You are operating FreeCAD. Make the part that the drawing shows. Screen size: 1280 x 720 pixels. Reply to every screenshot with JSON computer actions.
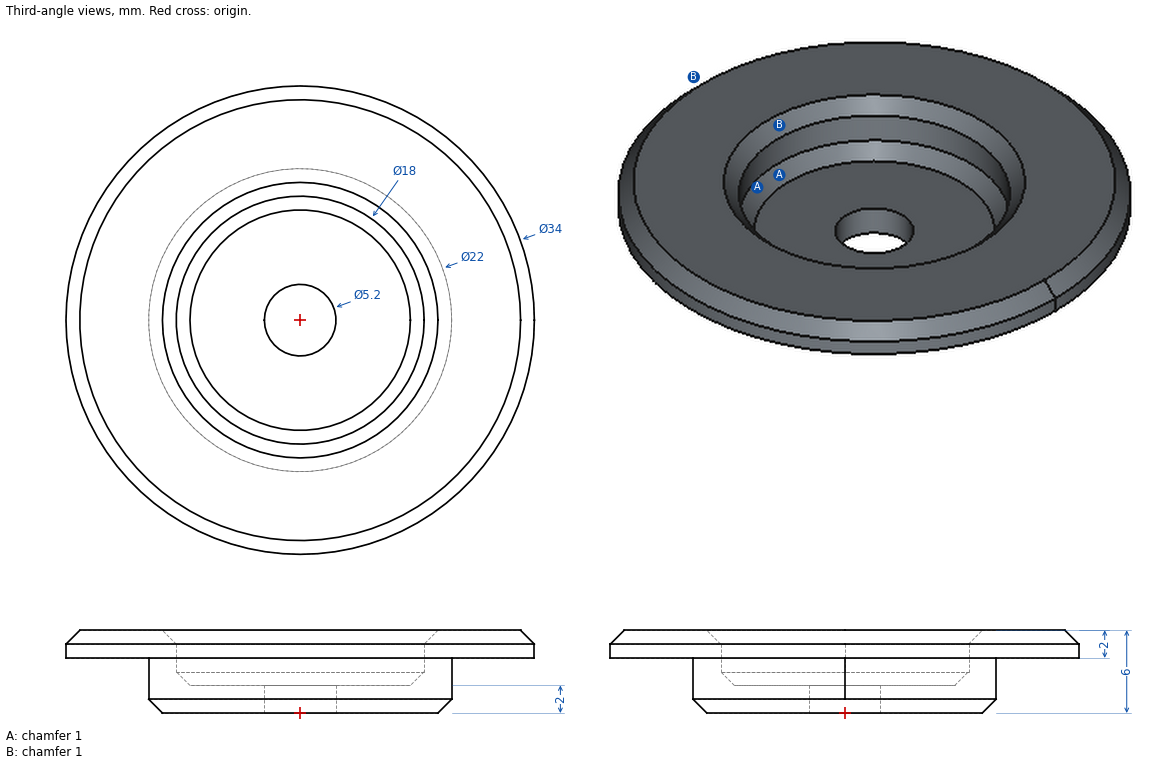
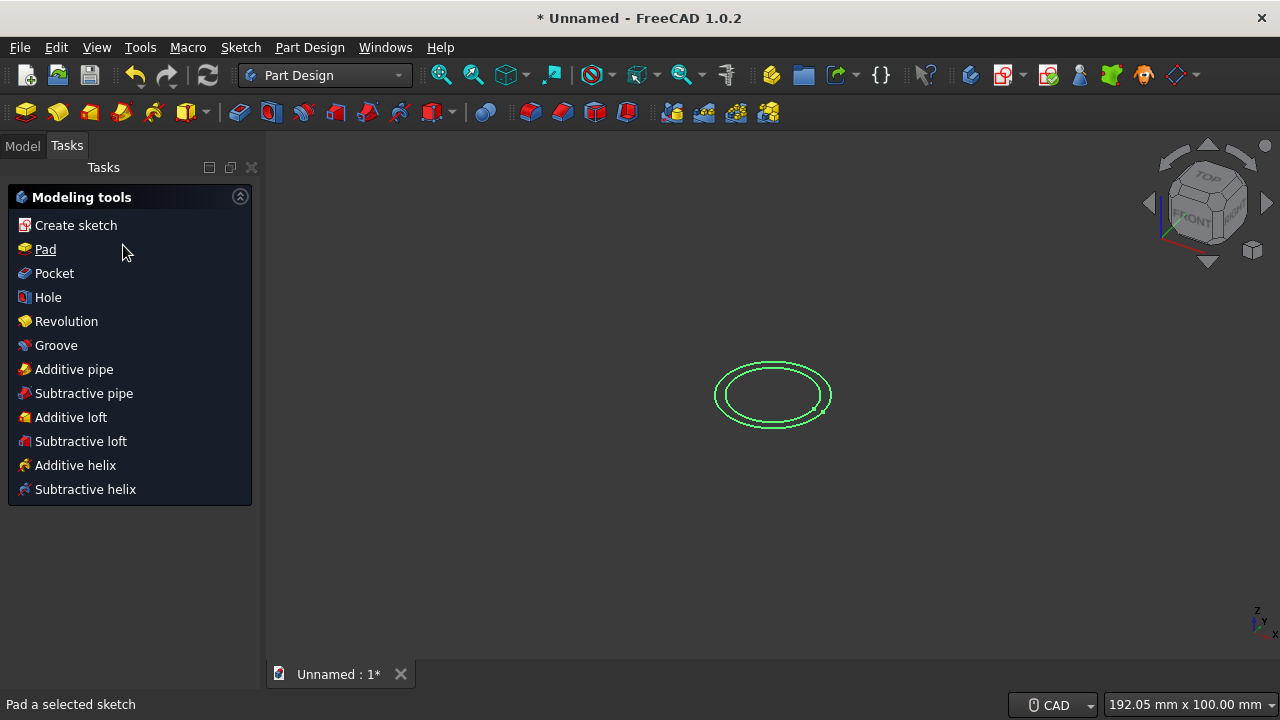
{"action": "left_click", "coordinate": [26, 112]}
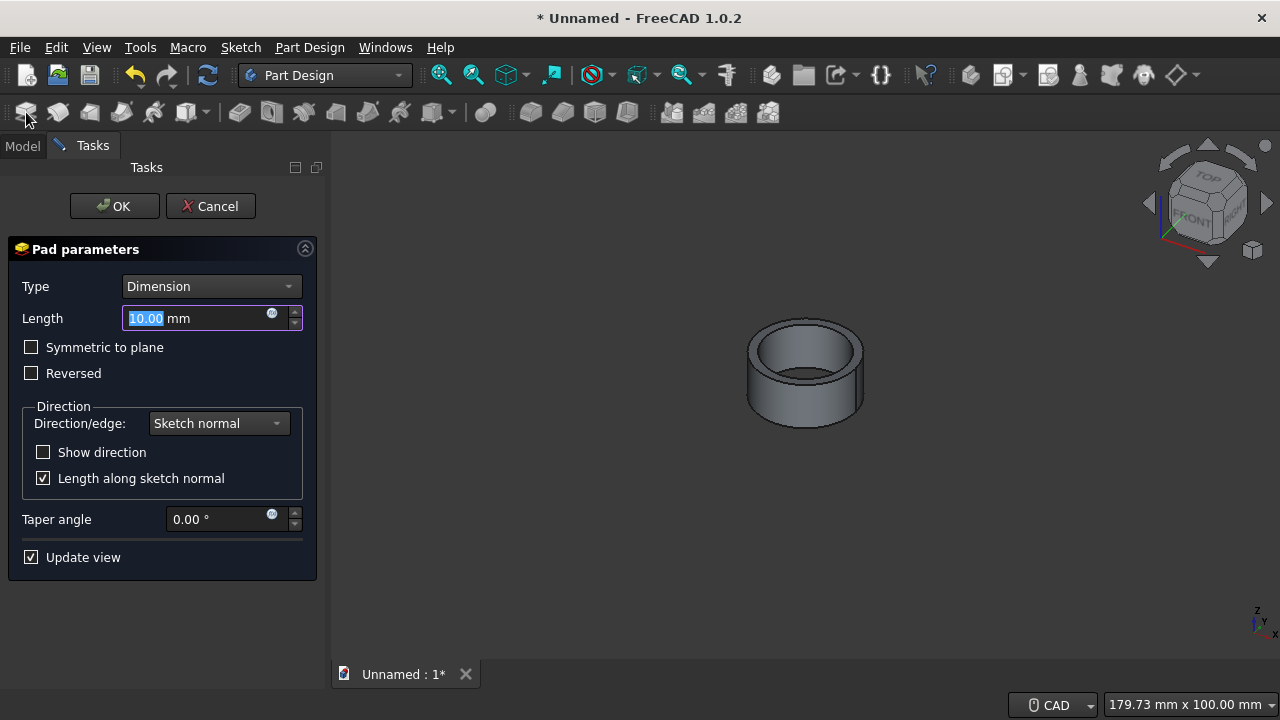
{"action": "type", "text": "6"}
{"action": "key", "text": "Tab"}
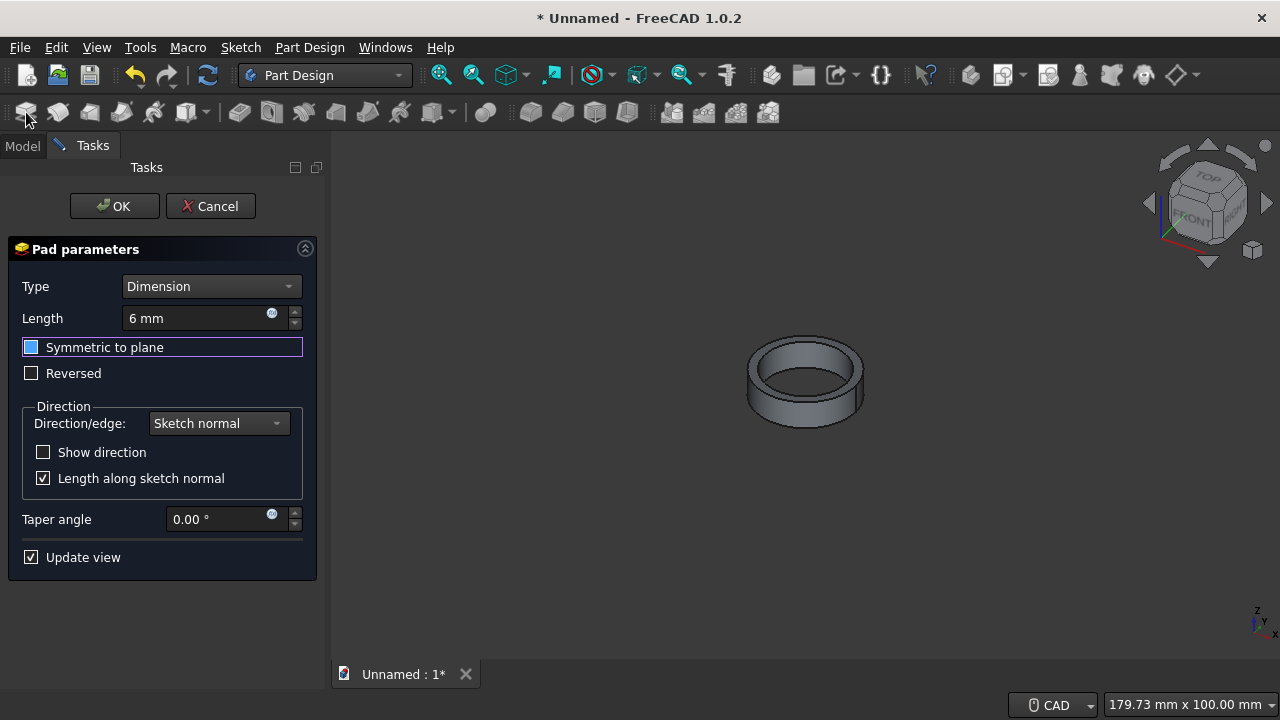
{"action": "left_click", "coordinate": [115, 206]}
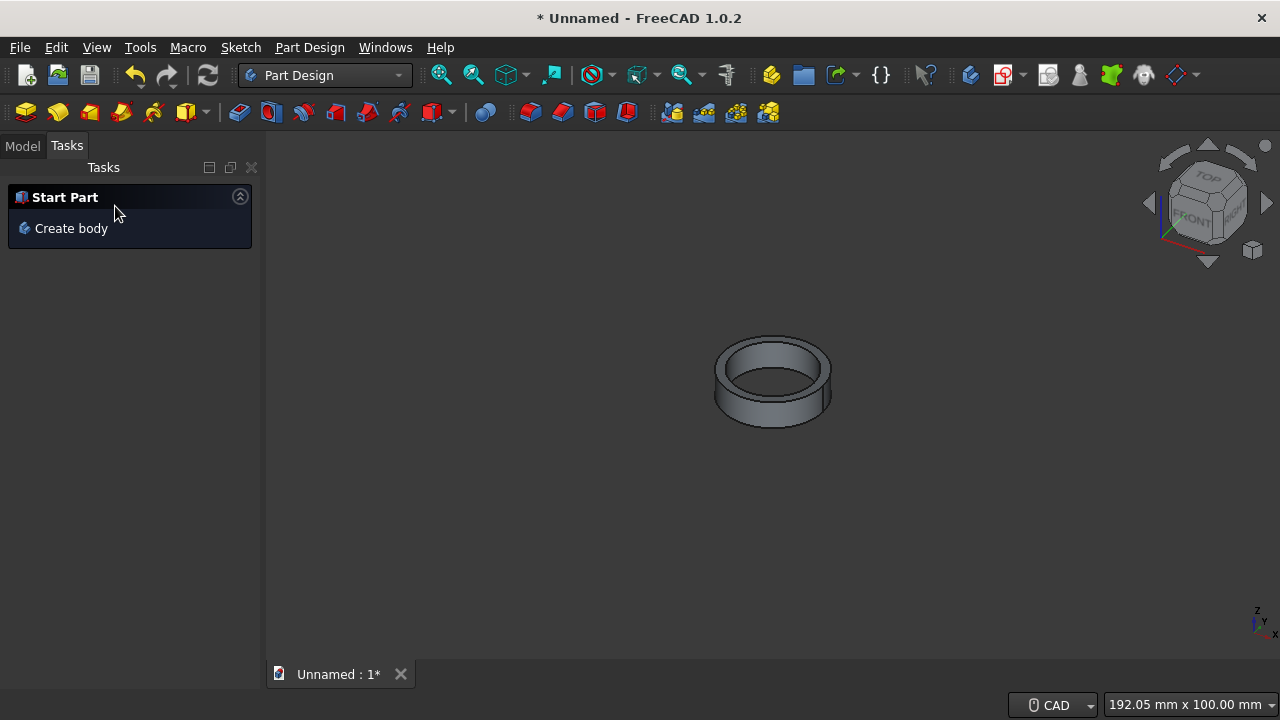
{"action": "left_click", "coordinate": [442, 76]}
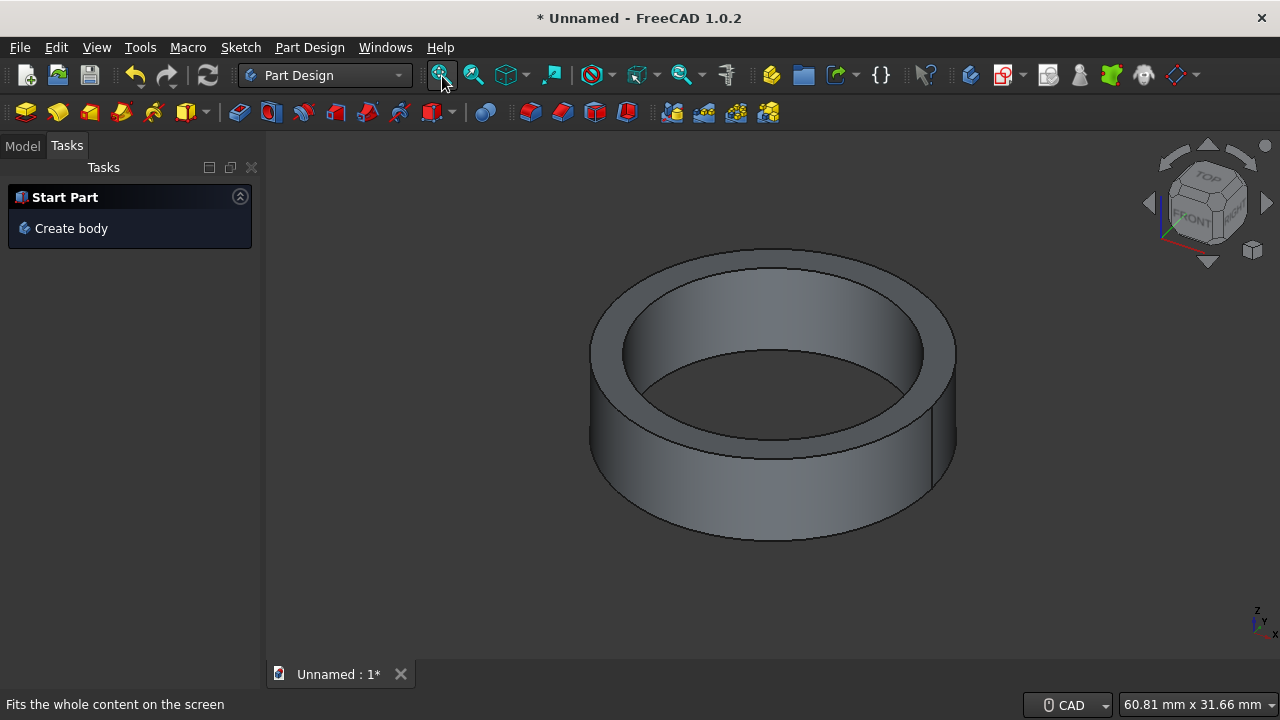
{"action": "key", "text": "5"}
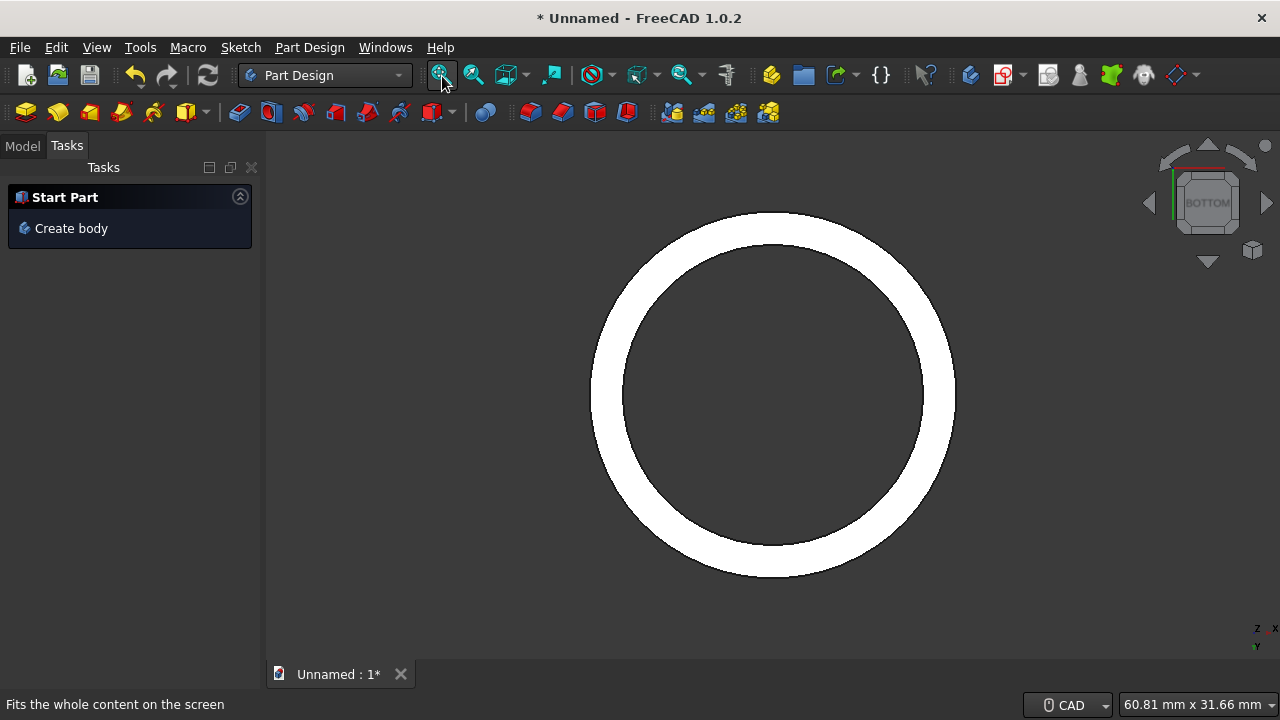
{"action": "left_click", "coordinate": [721, 237]}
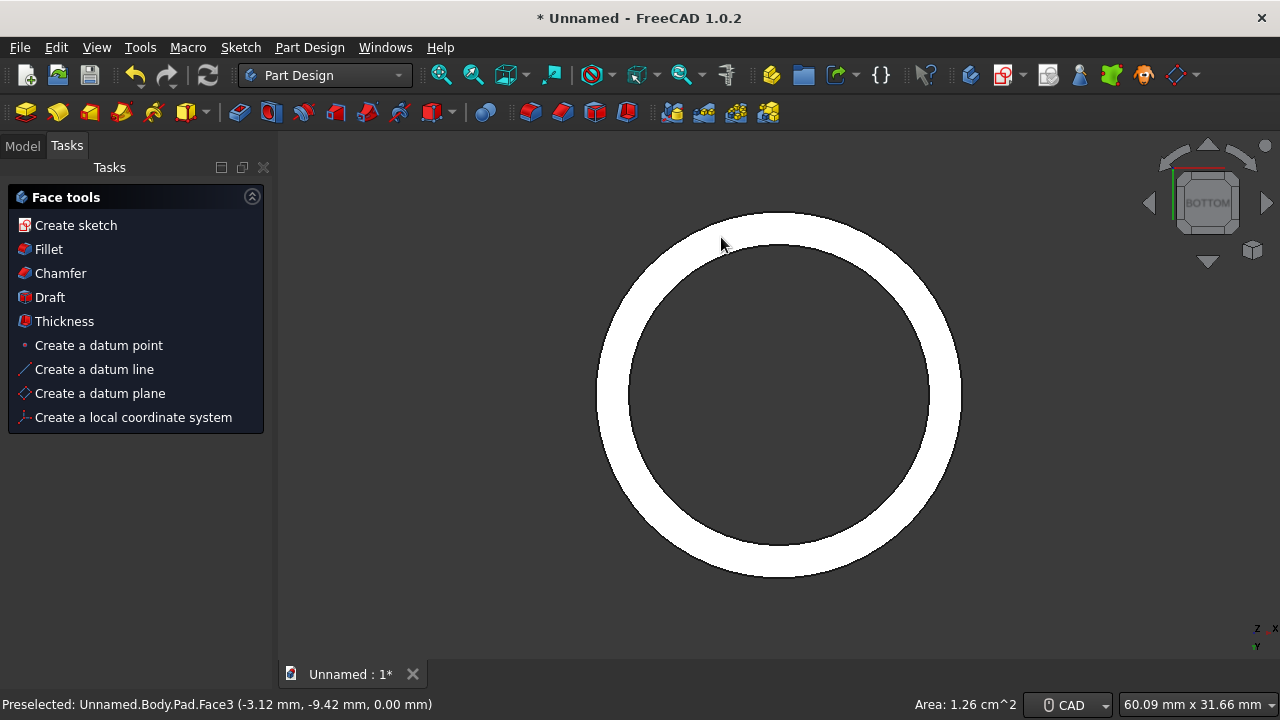
{"action": "left_click", "coordinate": [1004, 76]}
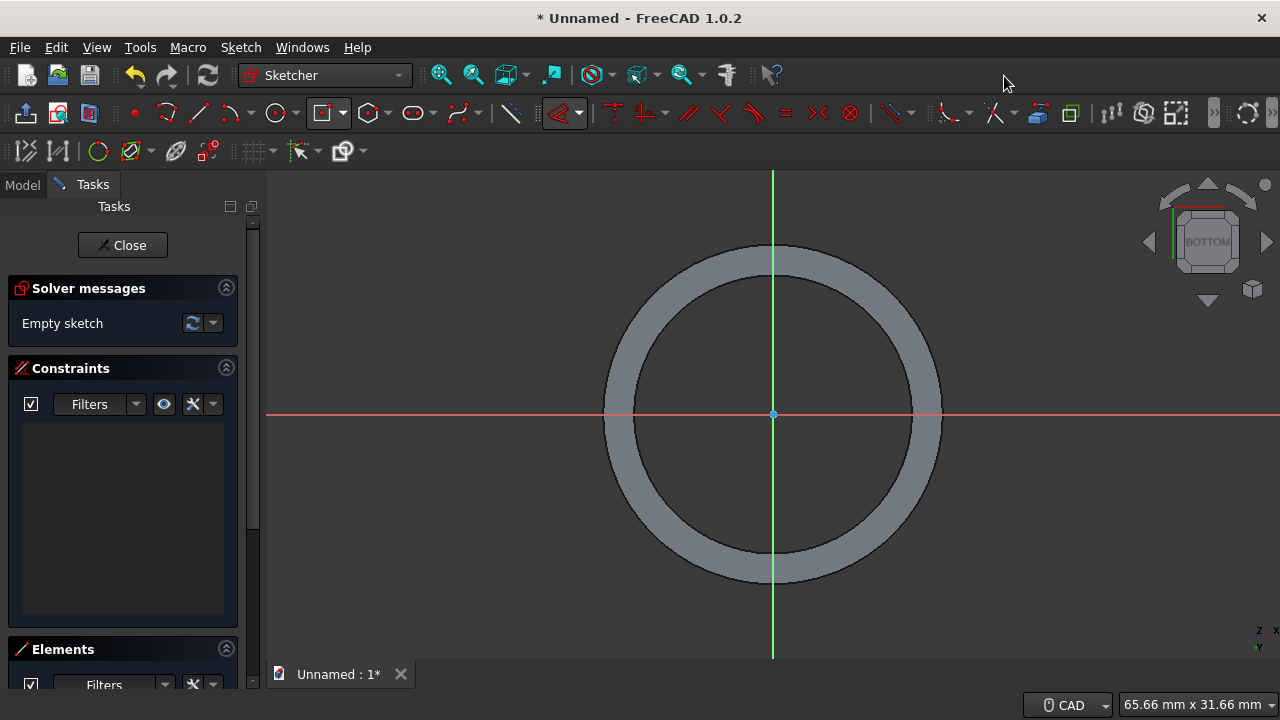
{"action": "key", "text": "g c"}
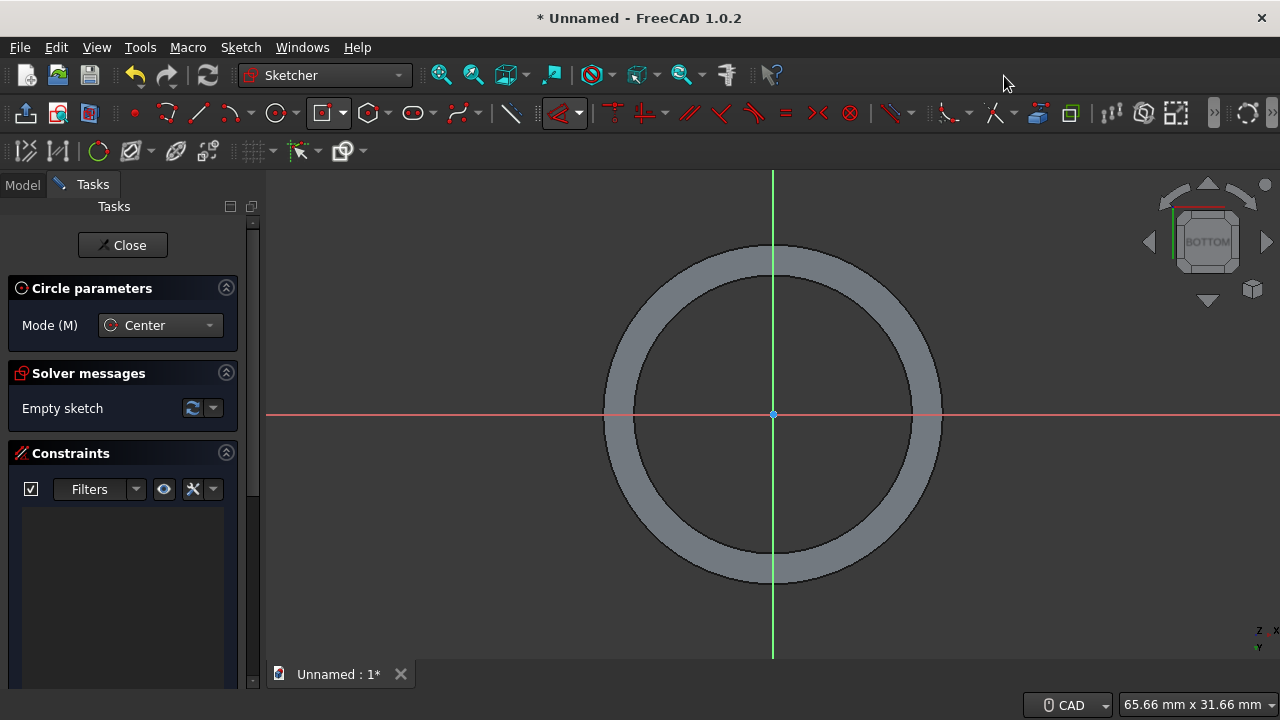
{"action": "left_click", "coordinate": [773, 414]}
{"action": "mouse_move", "coordinate": [893, 294]}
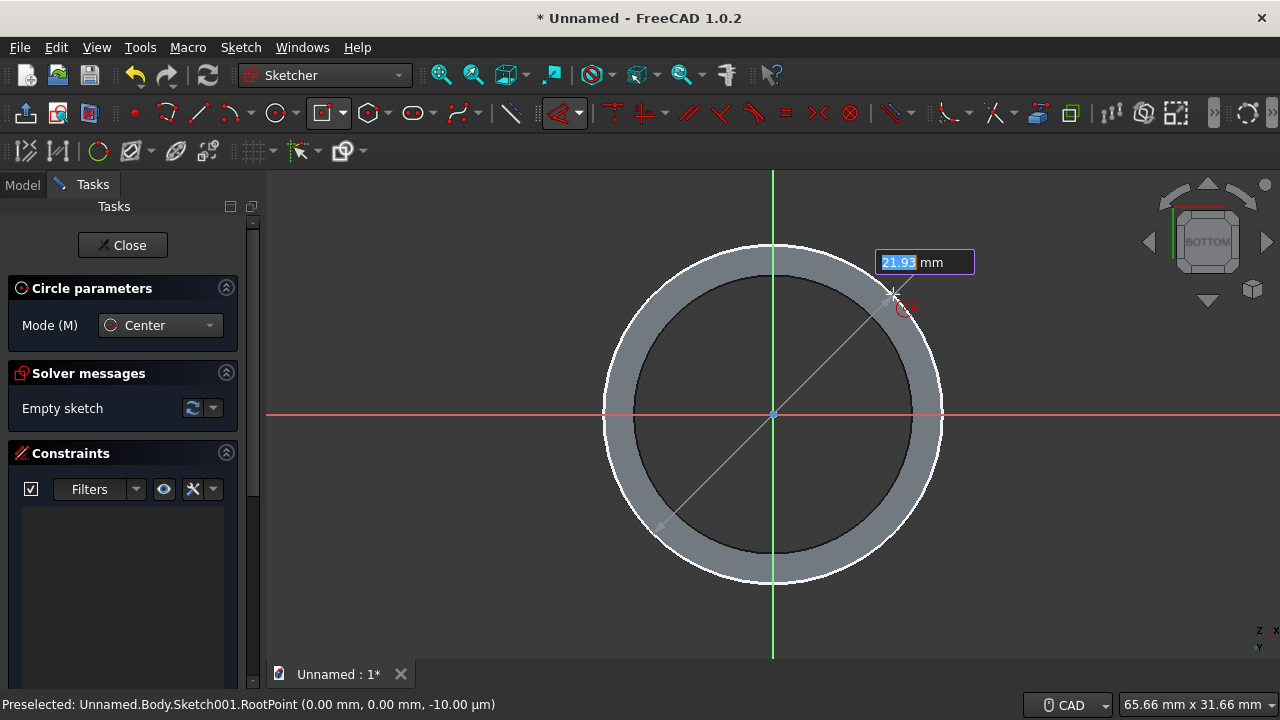
{"action": "type", "text": "22"}
{"action": "key", "text": "Return"}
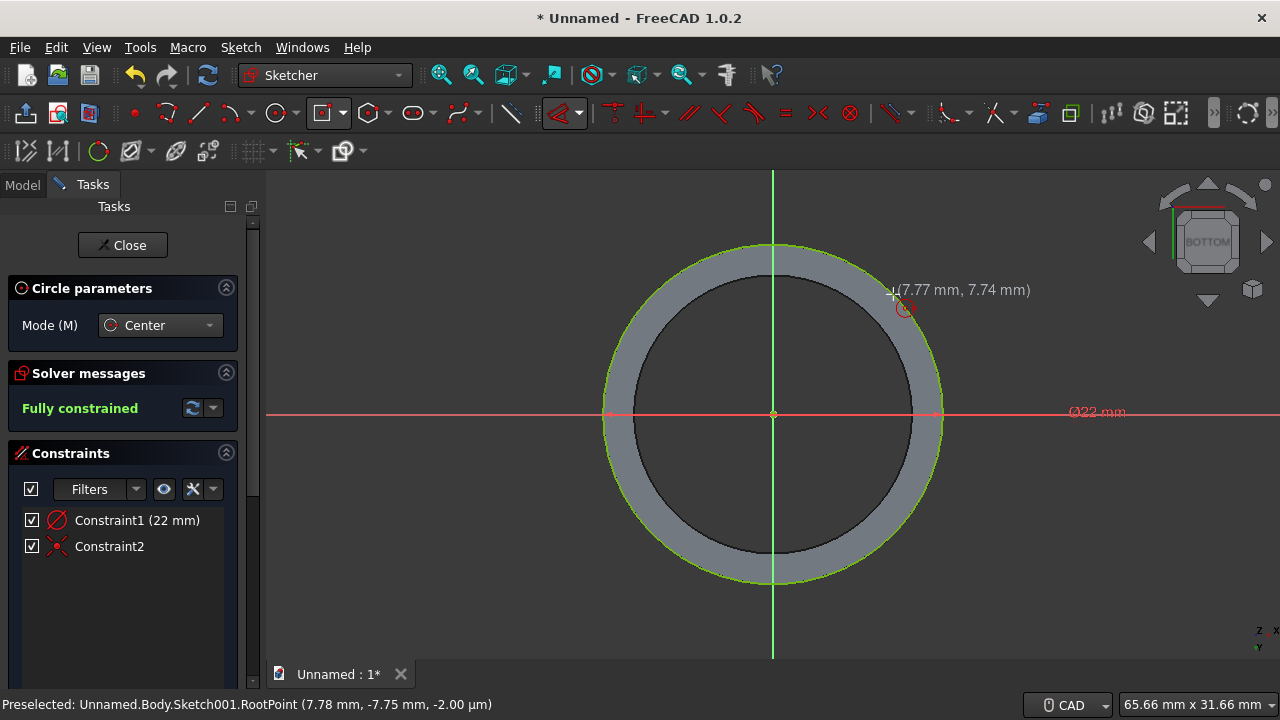
{"action": "left_click", "coordinate": [773, 414]}
{"action": "mouse_move", "coordinate": [801, 386]}